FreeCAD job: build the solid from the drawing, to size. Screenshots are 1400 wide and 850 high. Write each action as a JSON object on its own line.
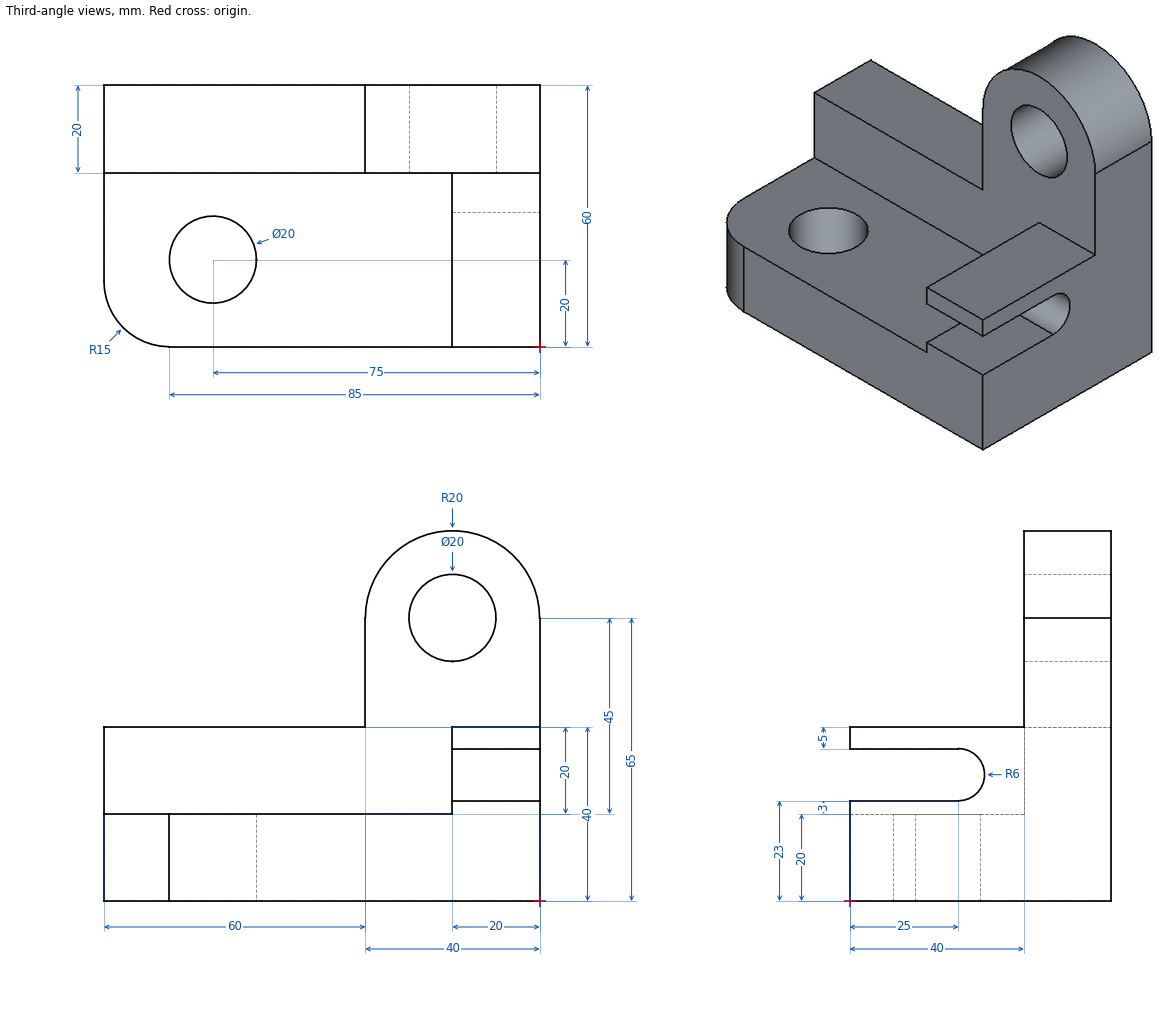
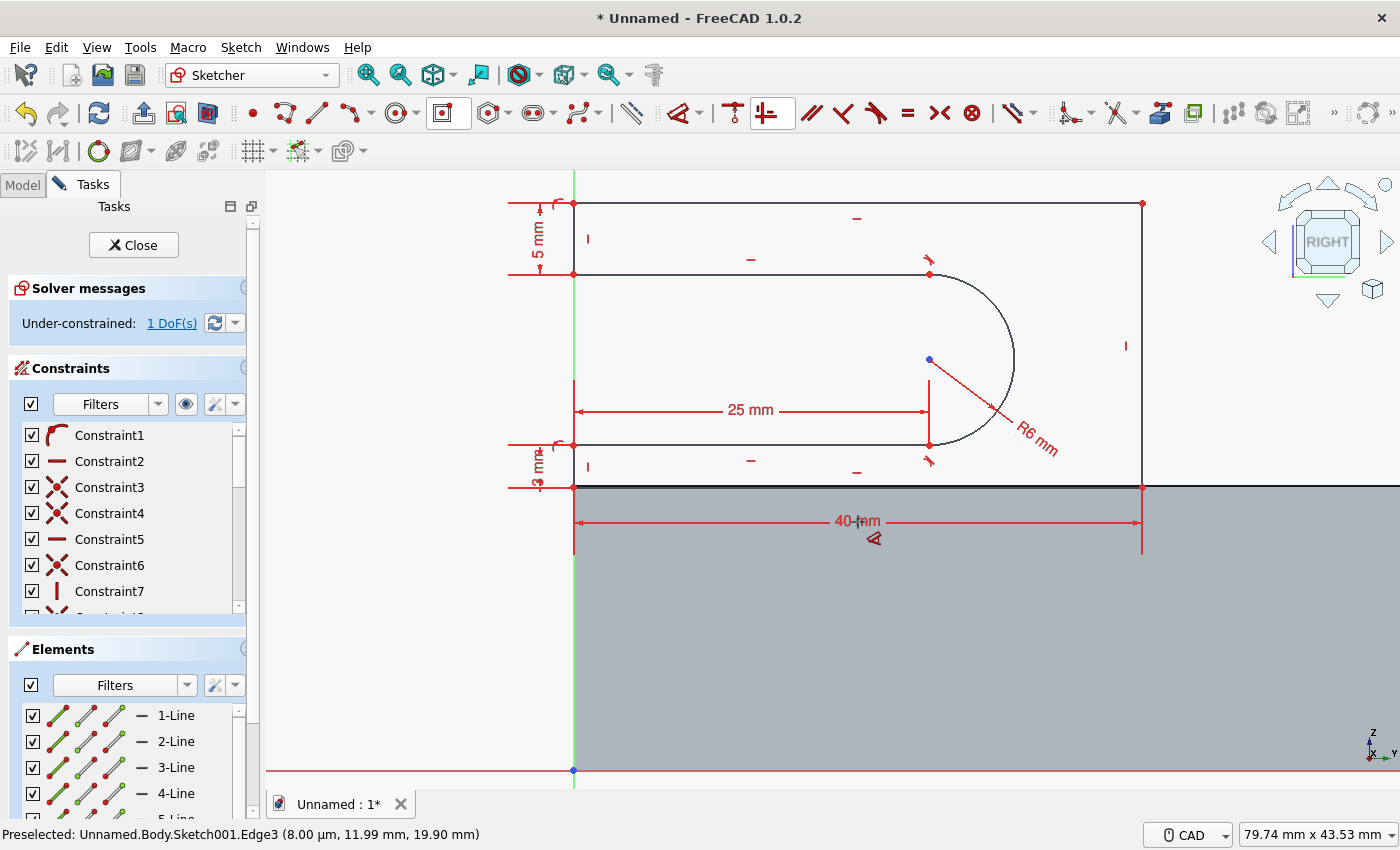
{"action": "left_click", "coordinate": [929, 445]}
{"action": "left_click", "coordinate": [540, 603]}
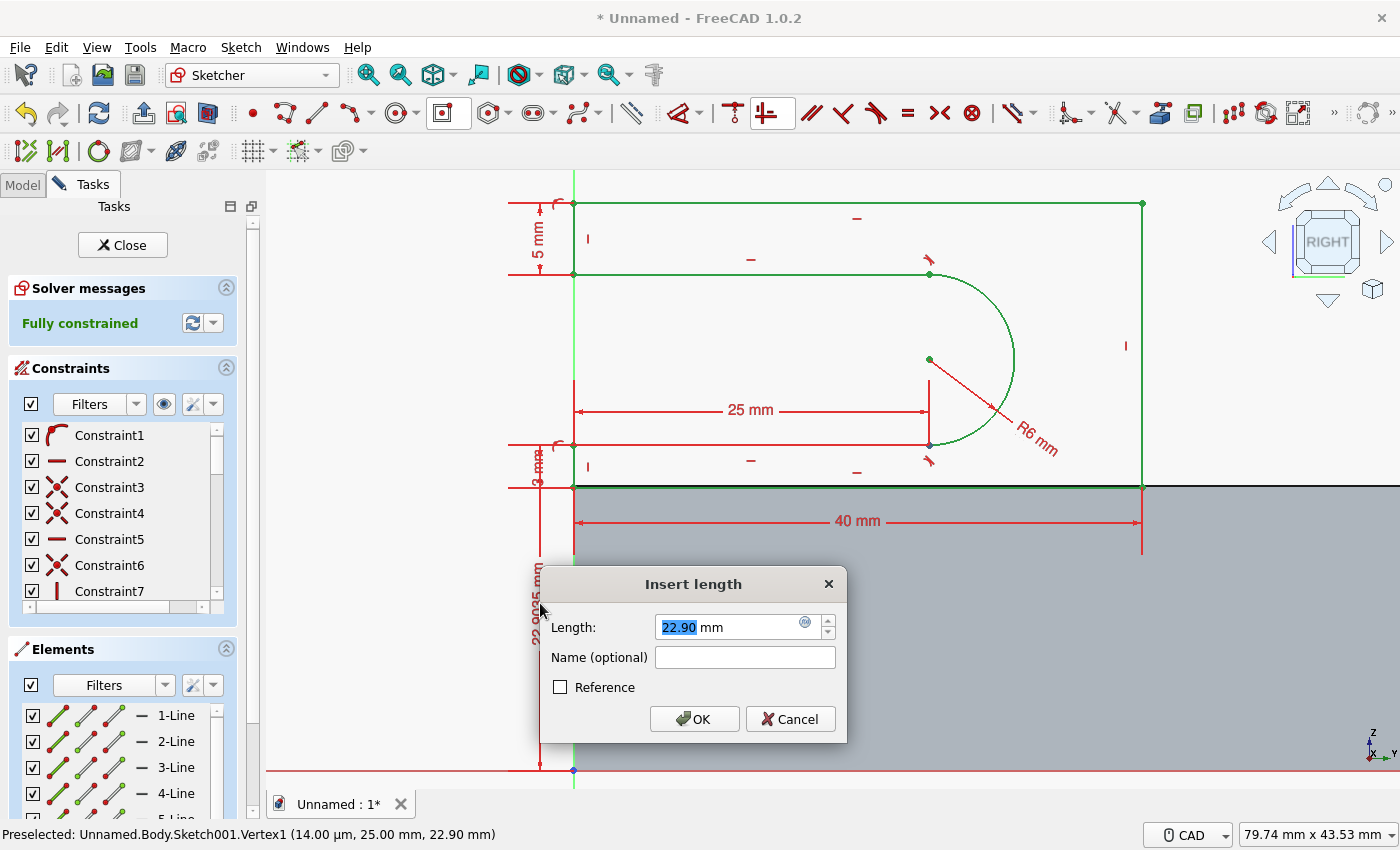
{"action": "type", "text": "23"}
{"action": "key", "text": "Return"}
{"action": "key", "text": "Escape"}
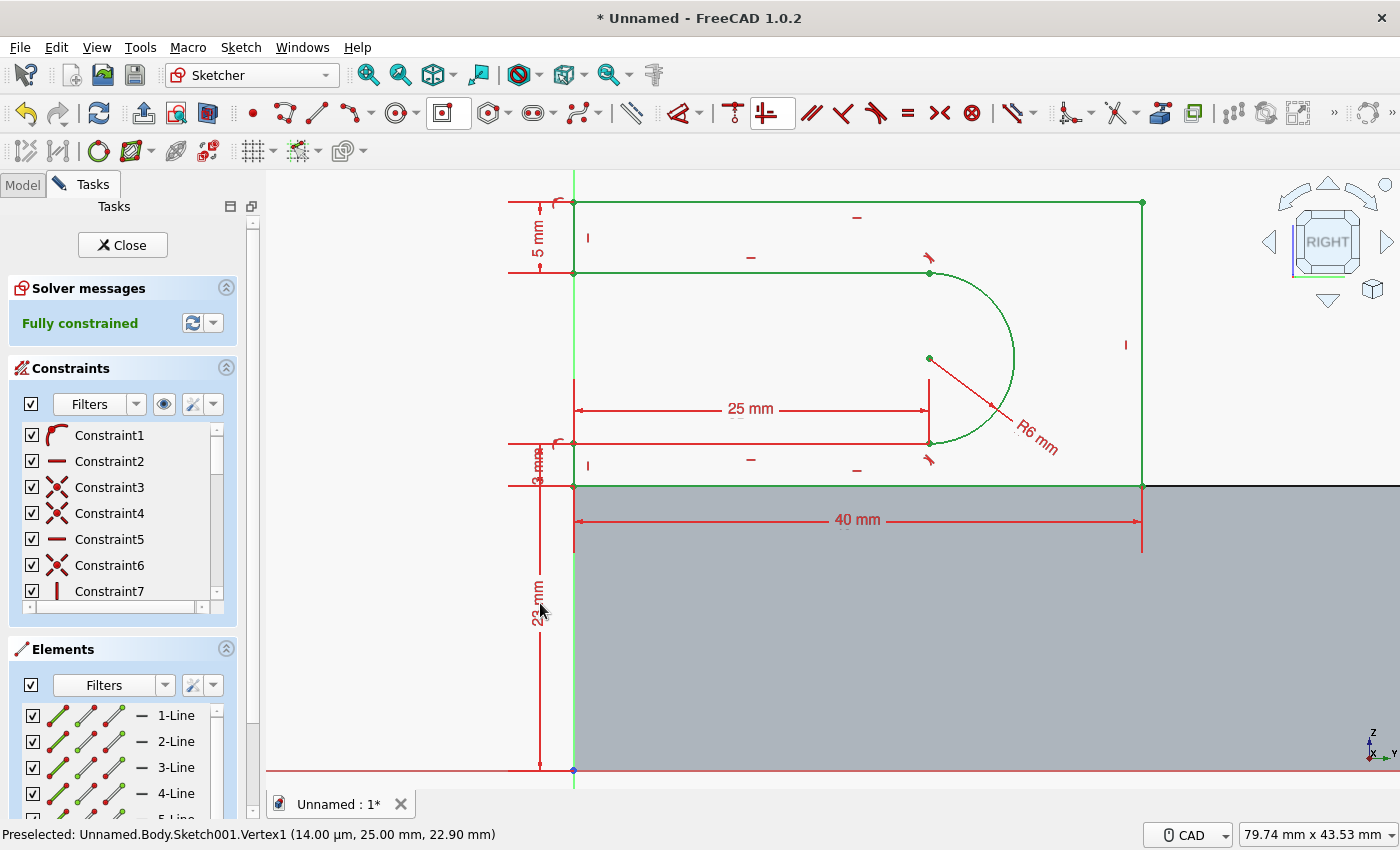
{"action": "left_click", "coordinate": [123, 245]}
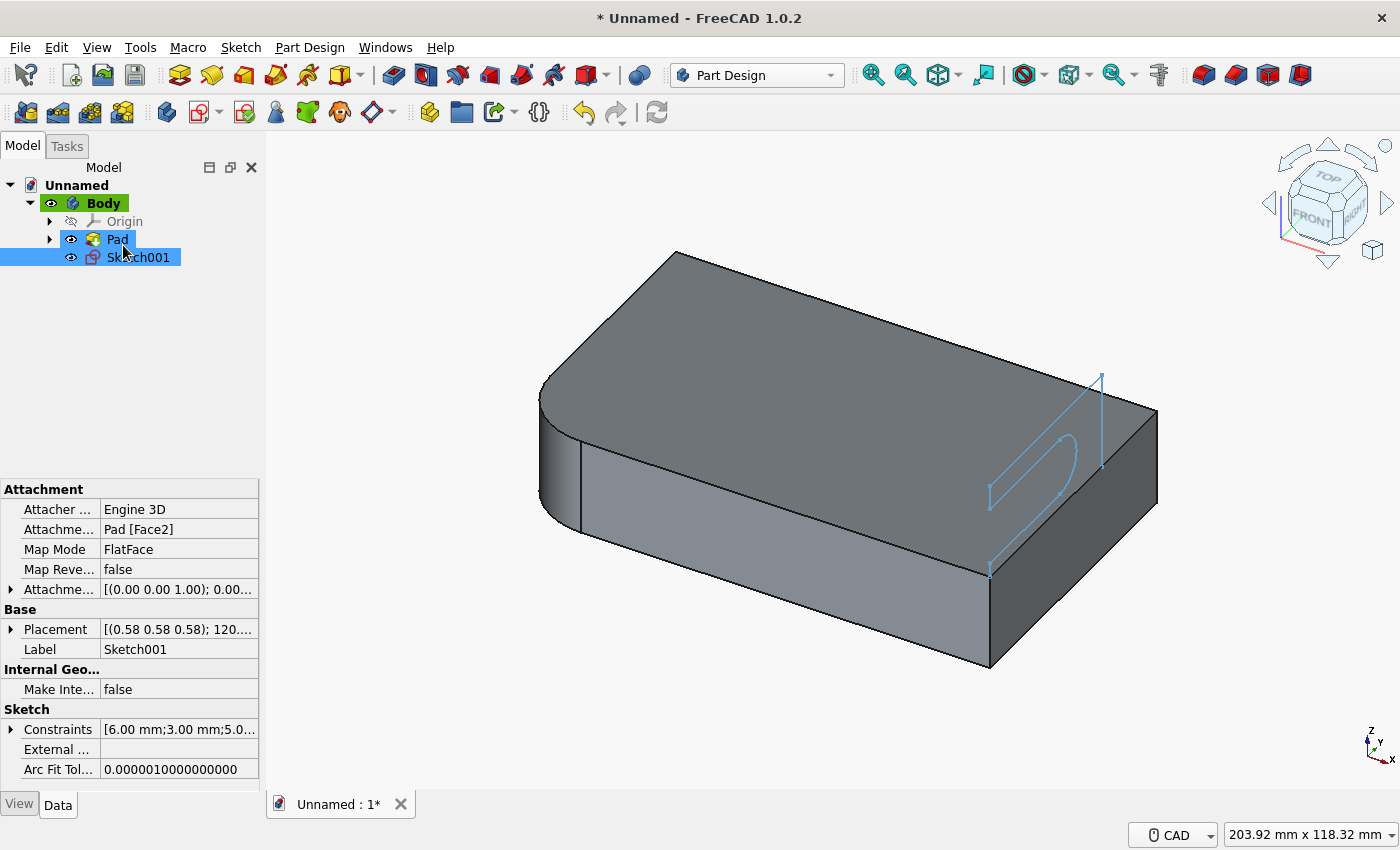
{"action": "left_click", "coordinate": [180, 76]}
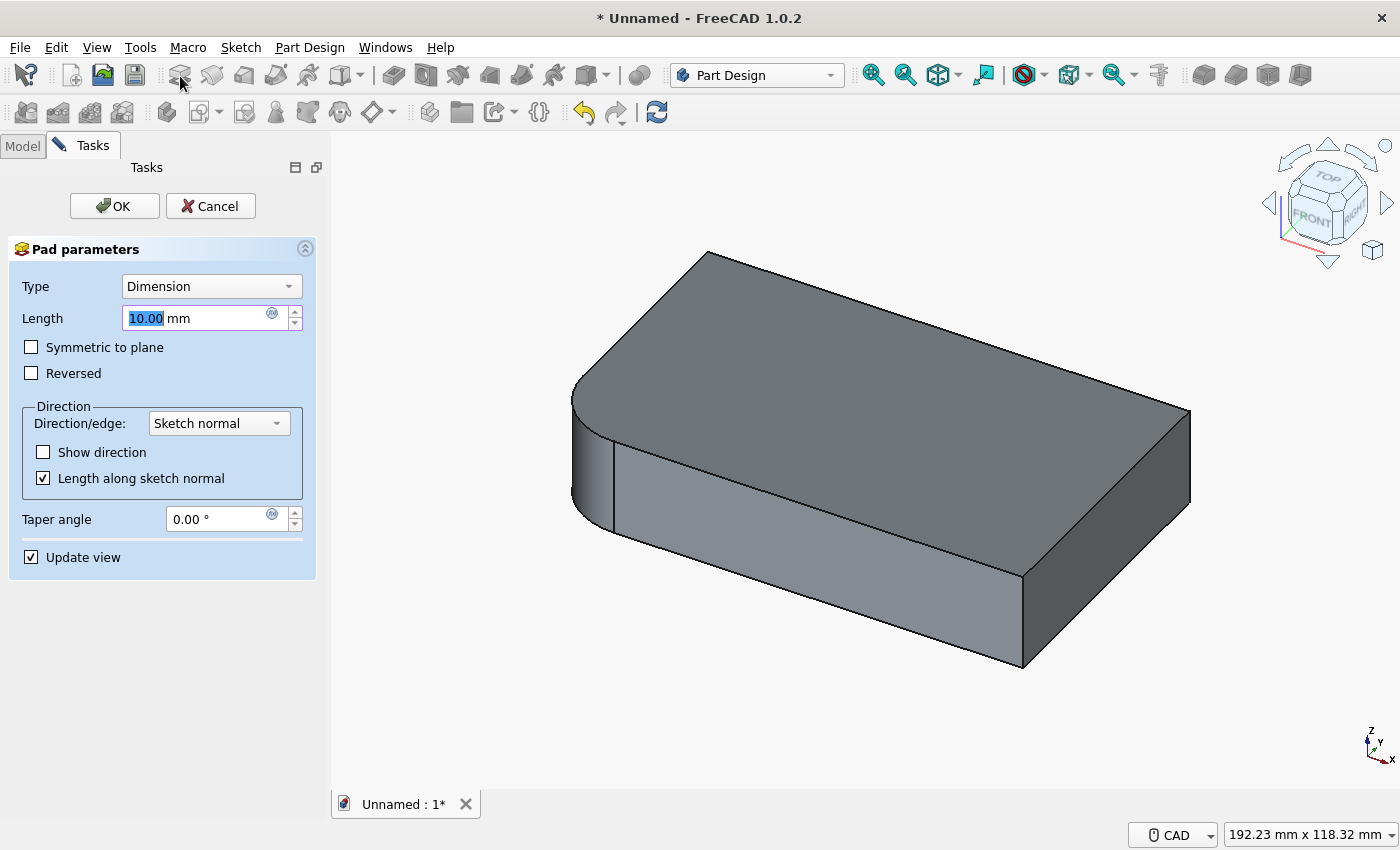
{"action": "type", "text": "20"}
{"action": "key", "text": "Tab"}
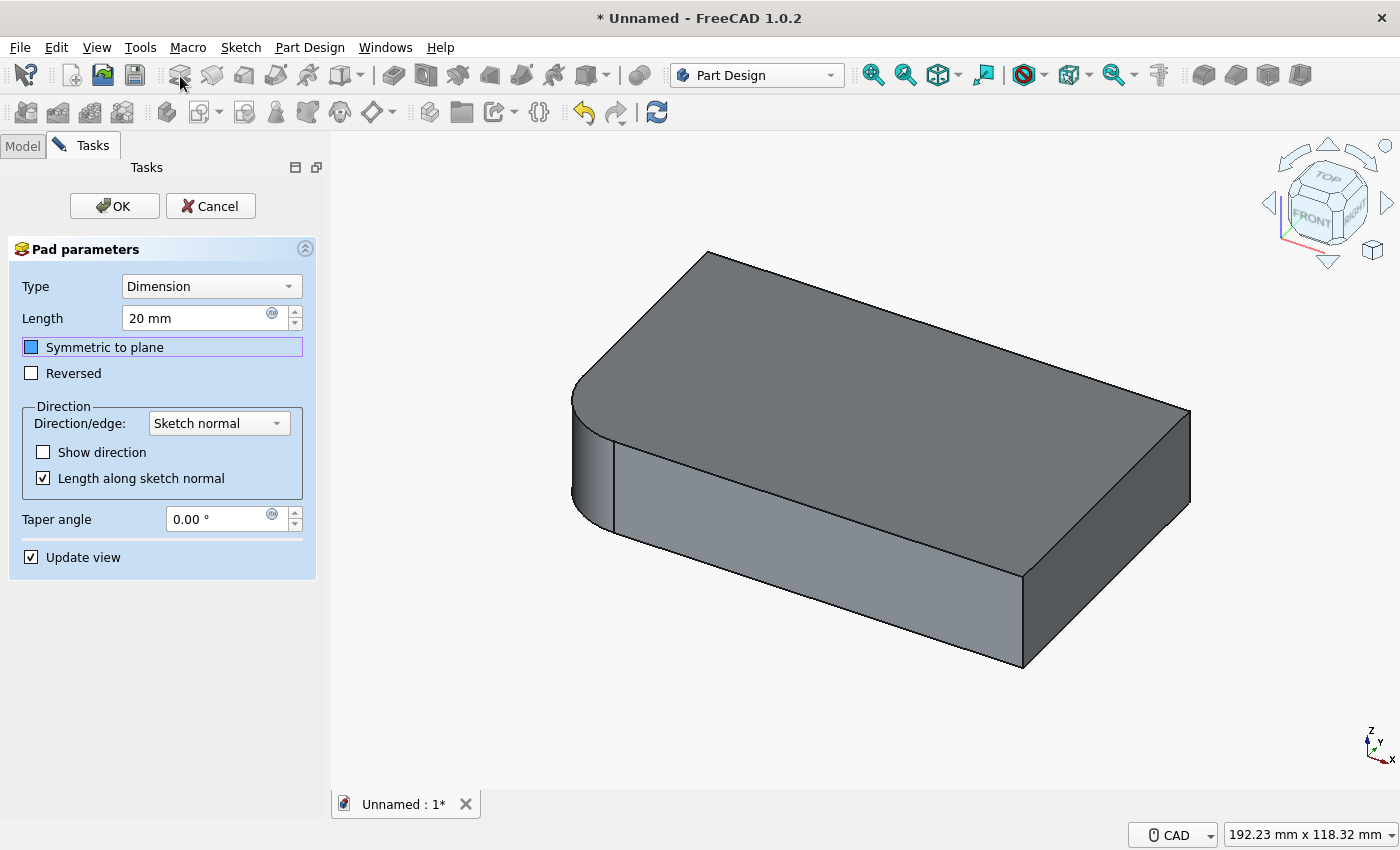
{"action": "left_click", "coordinate": [30, 373]}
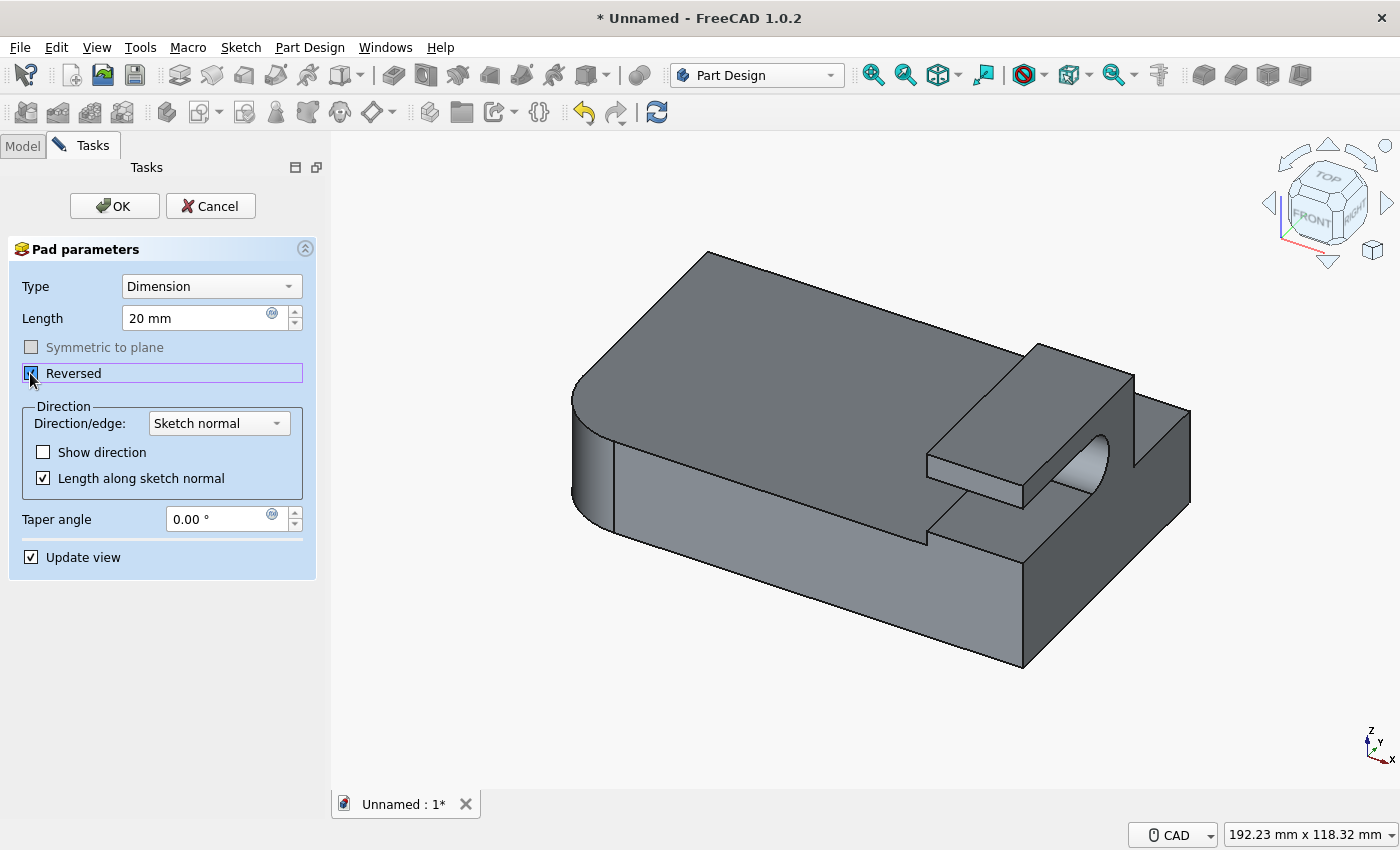
{"action": "left_click", "coordinate": [115, 206]}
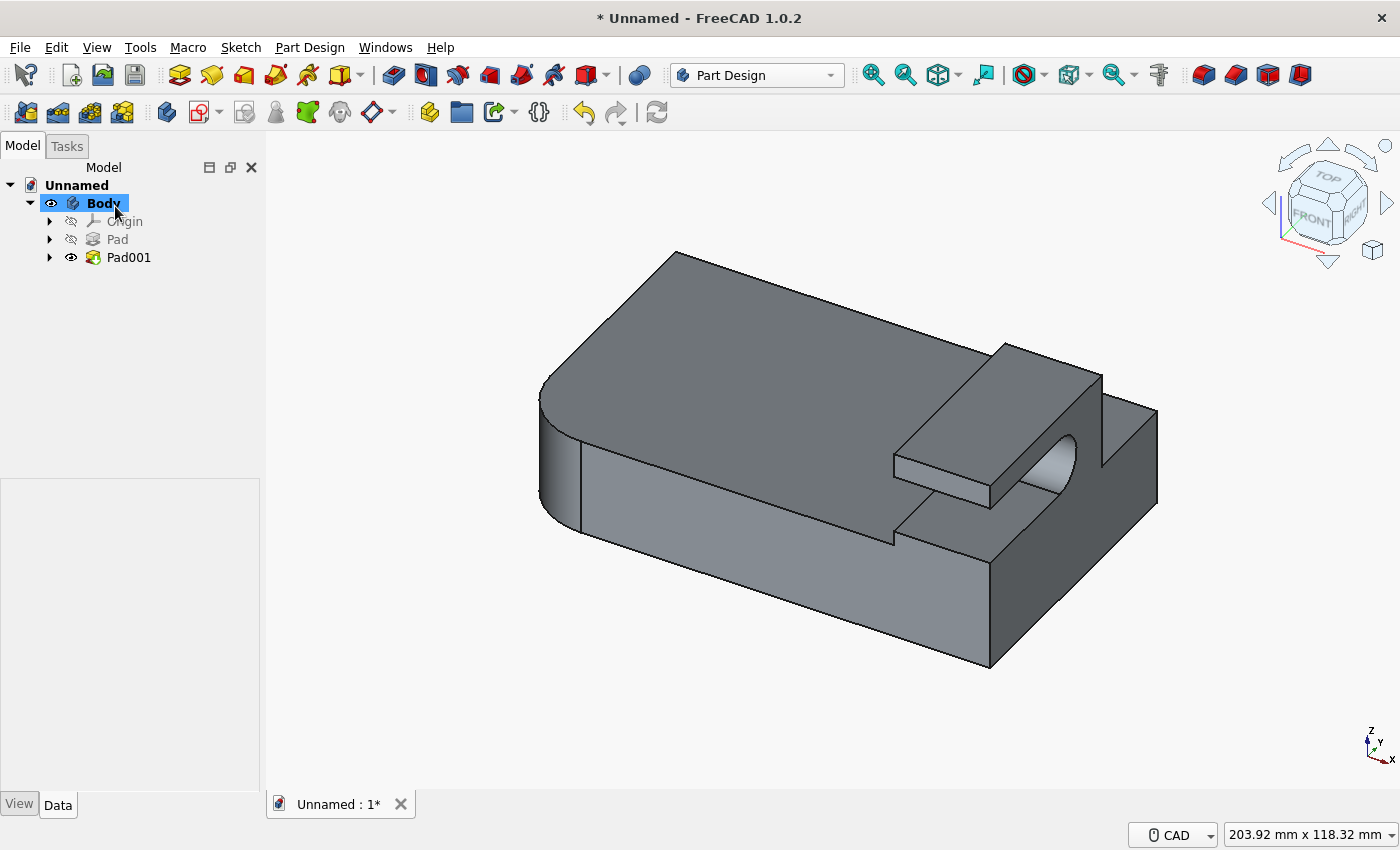
{"action": "key", "text": "4"}